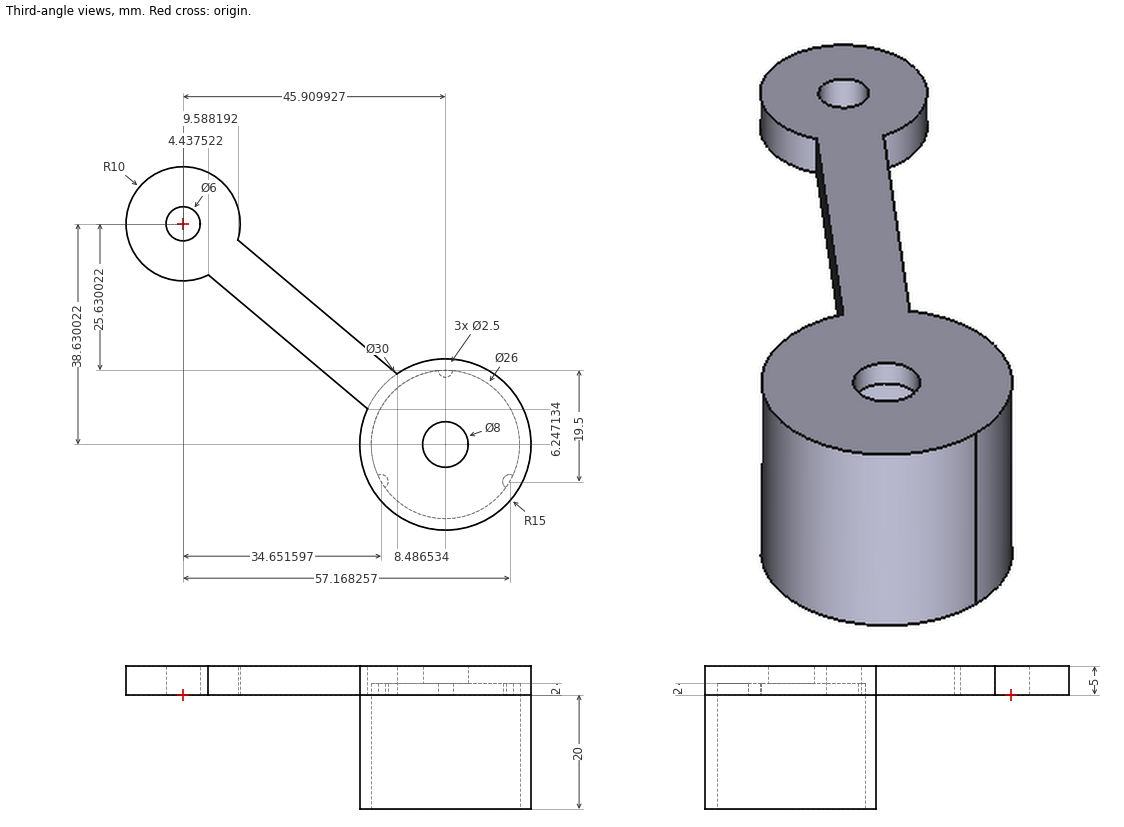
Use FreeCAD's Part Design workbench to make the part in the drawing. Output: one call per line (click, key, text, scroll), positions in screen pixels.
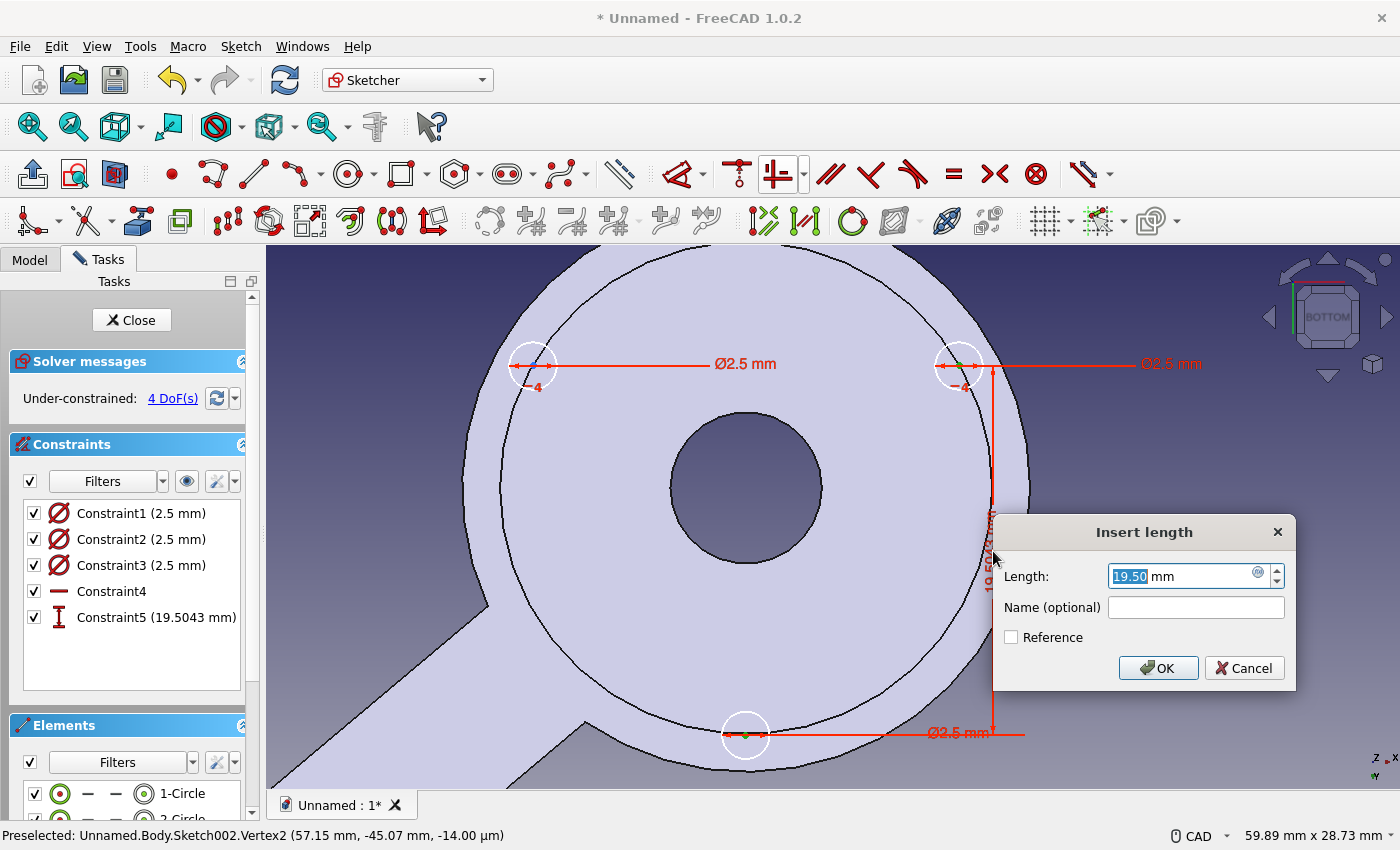
text(19.5)
key(Return)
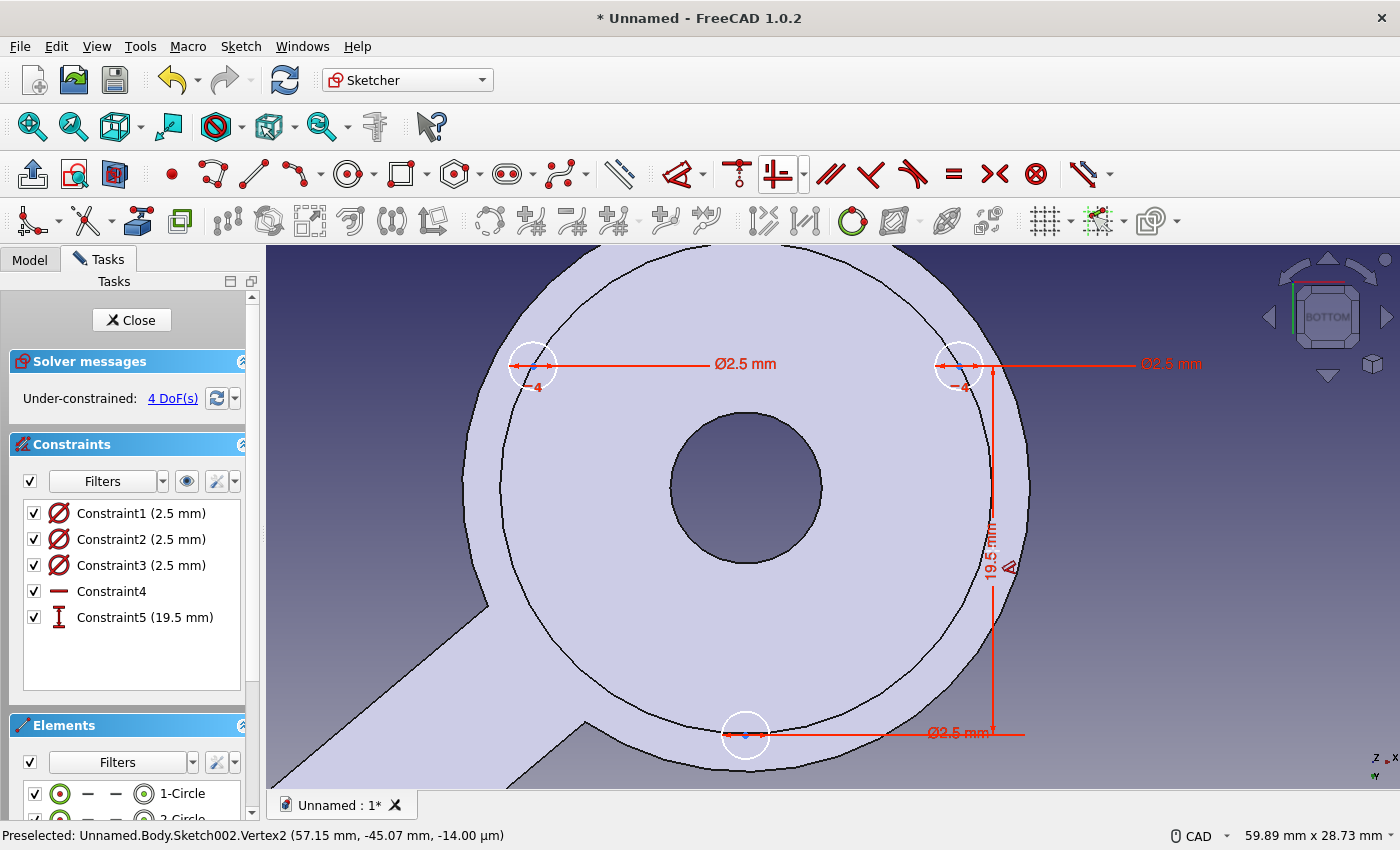
click(746, 735)
click(520, 701)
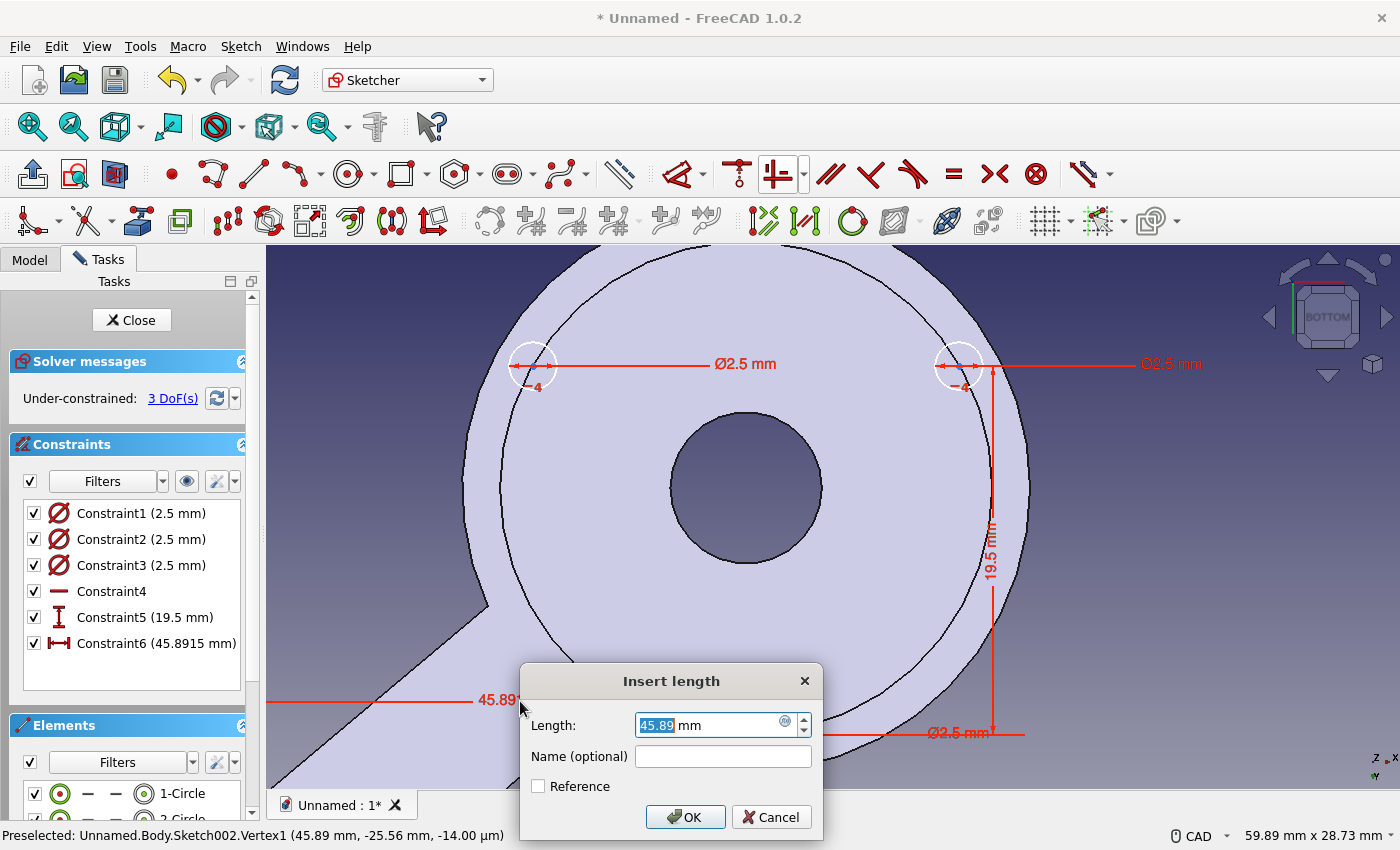
text(45.909927)
key(Return)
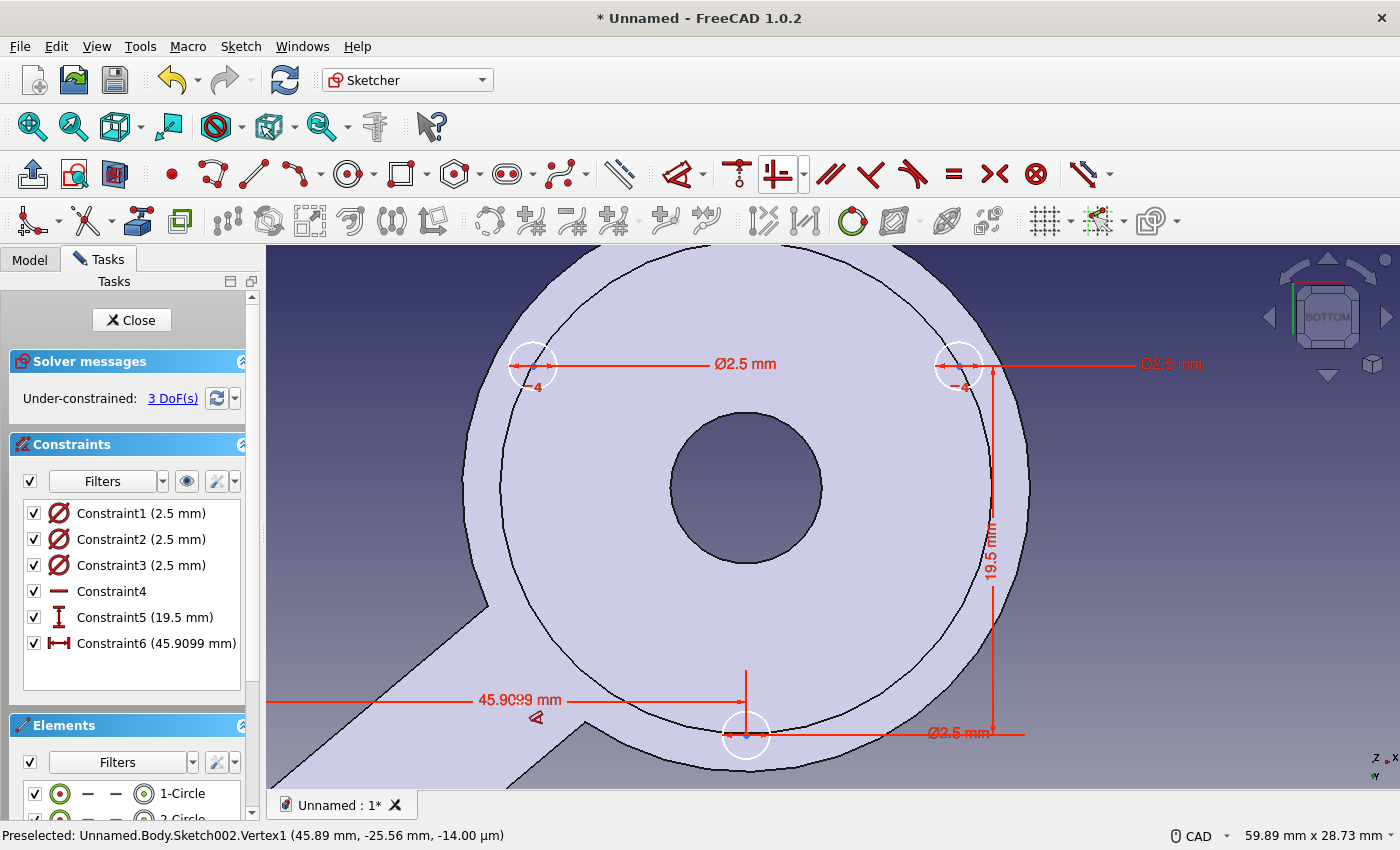
click(746, 735)
click(780, 754)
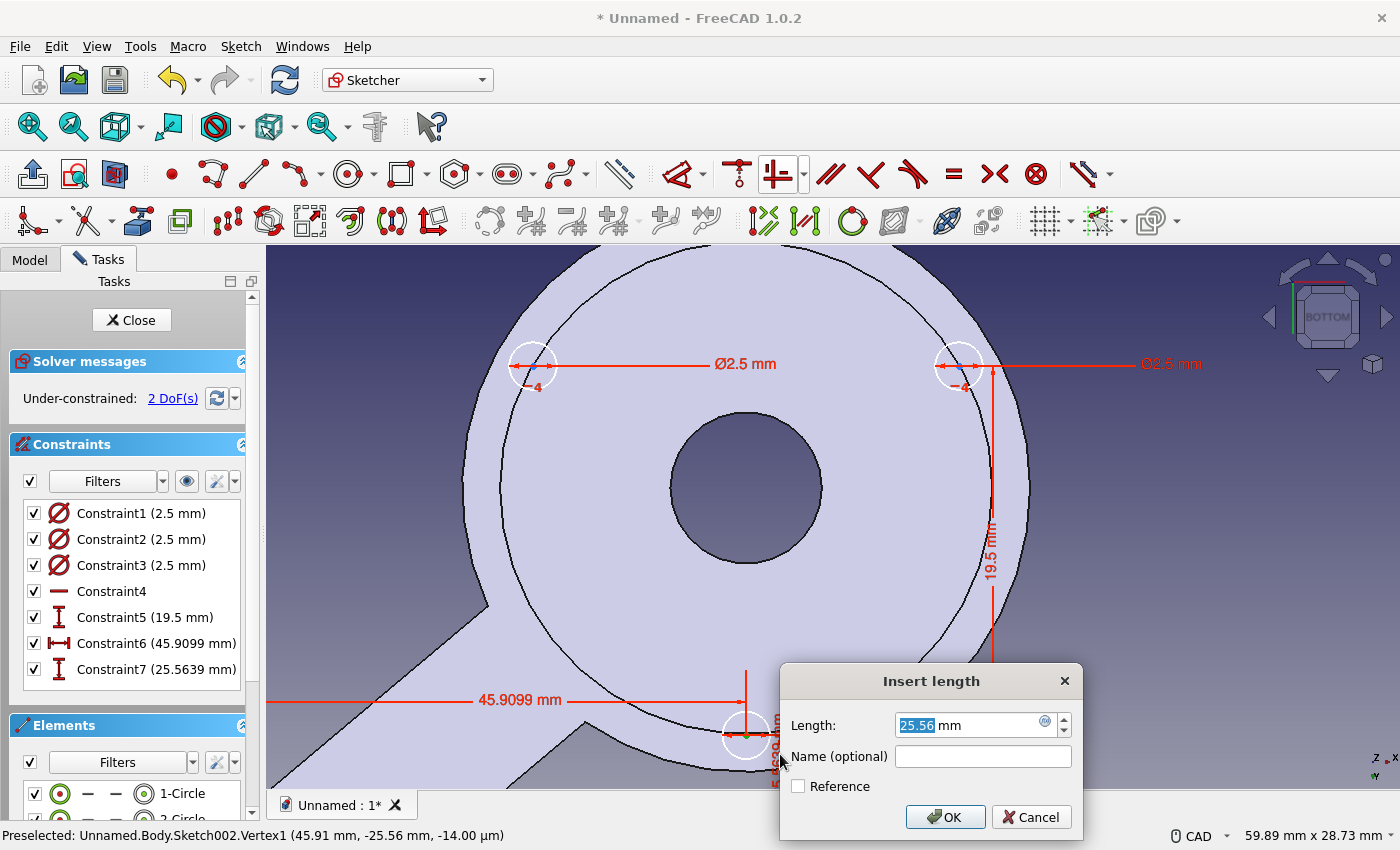
text(25.630022)
key(Return)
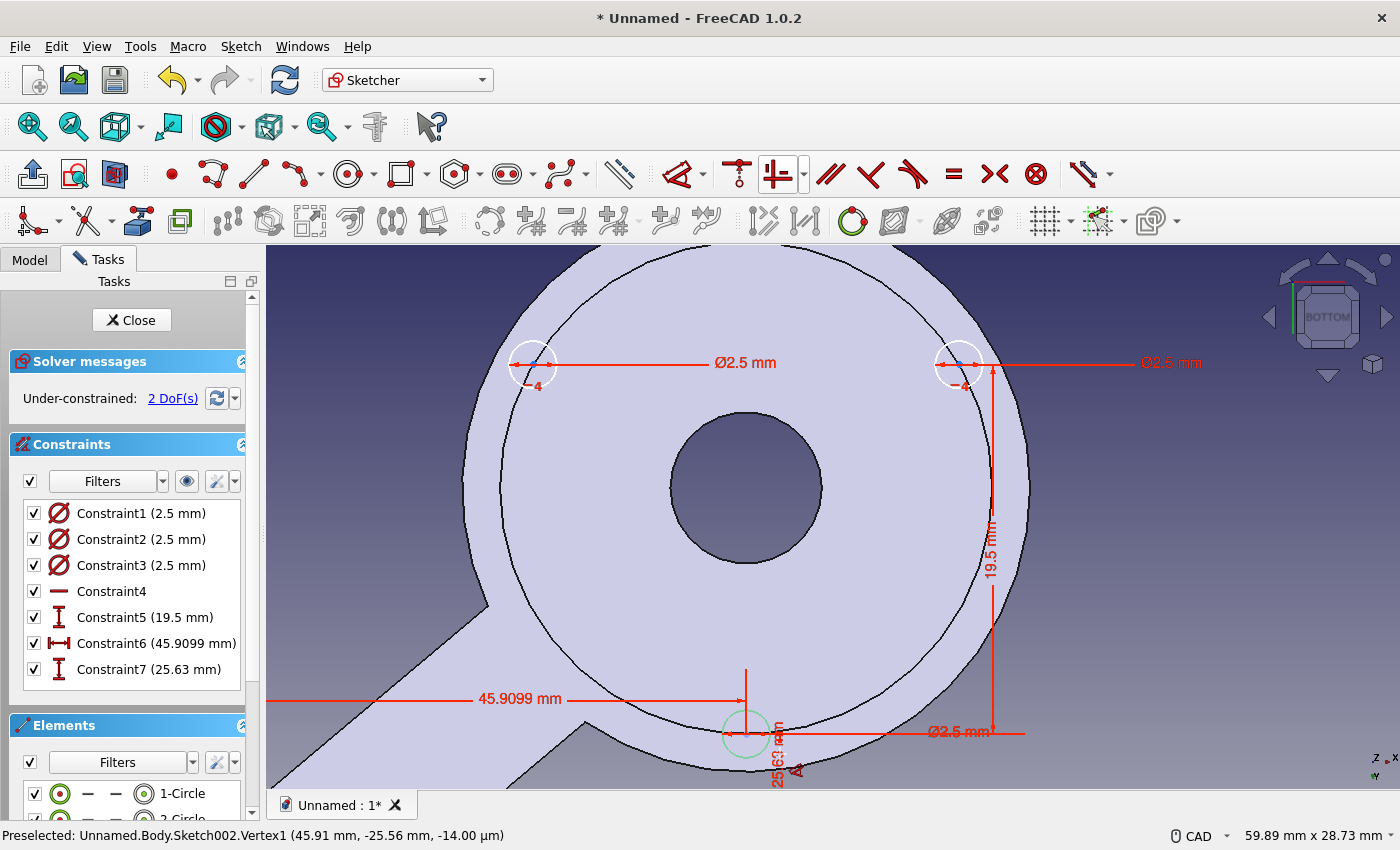
click(959, 365)
click(626, 331)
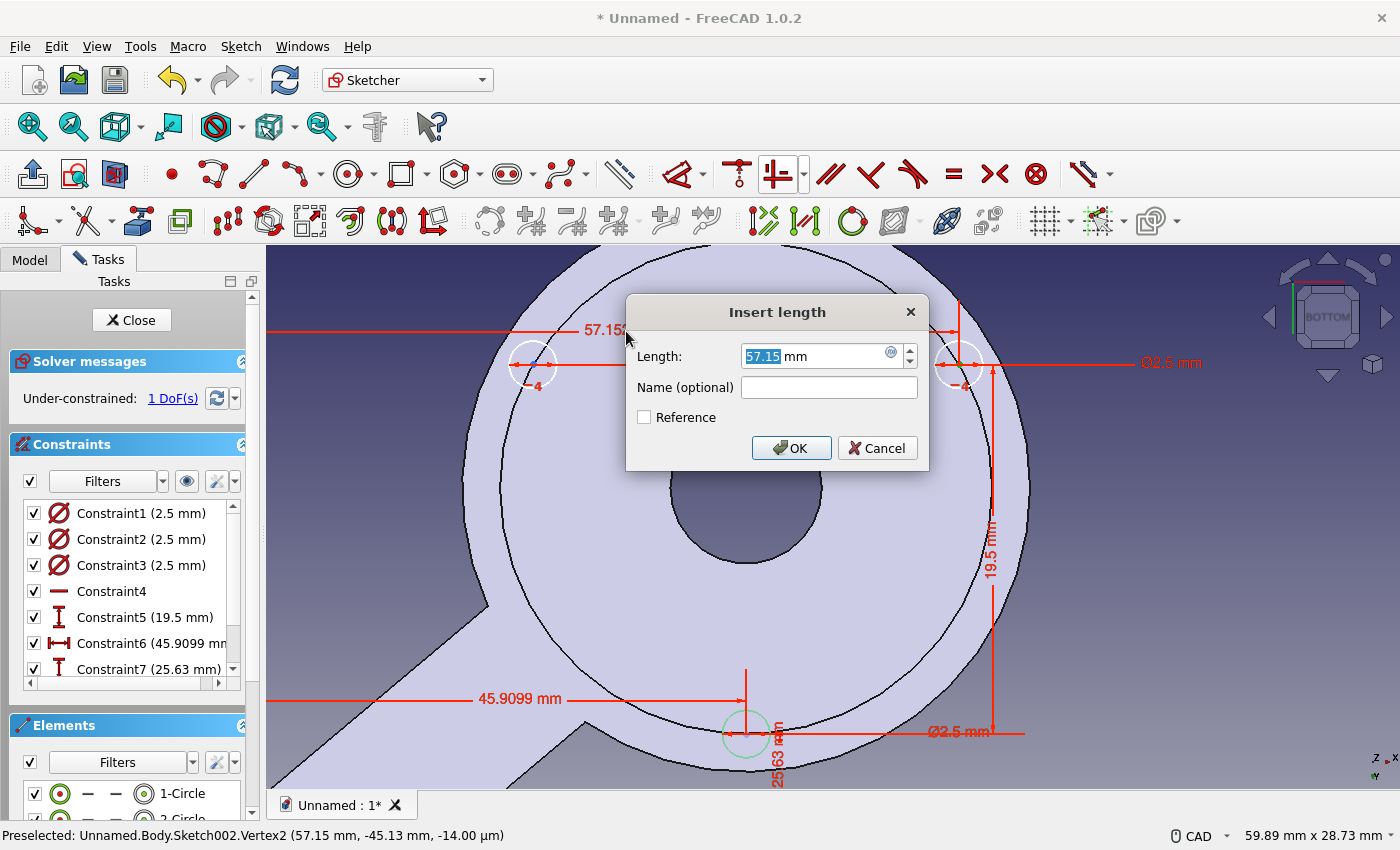
text(57.168257)
key(Return)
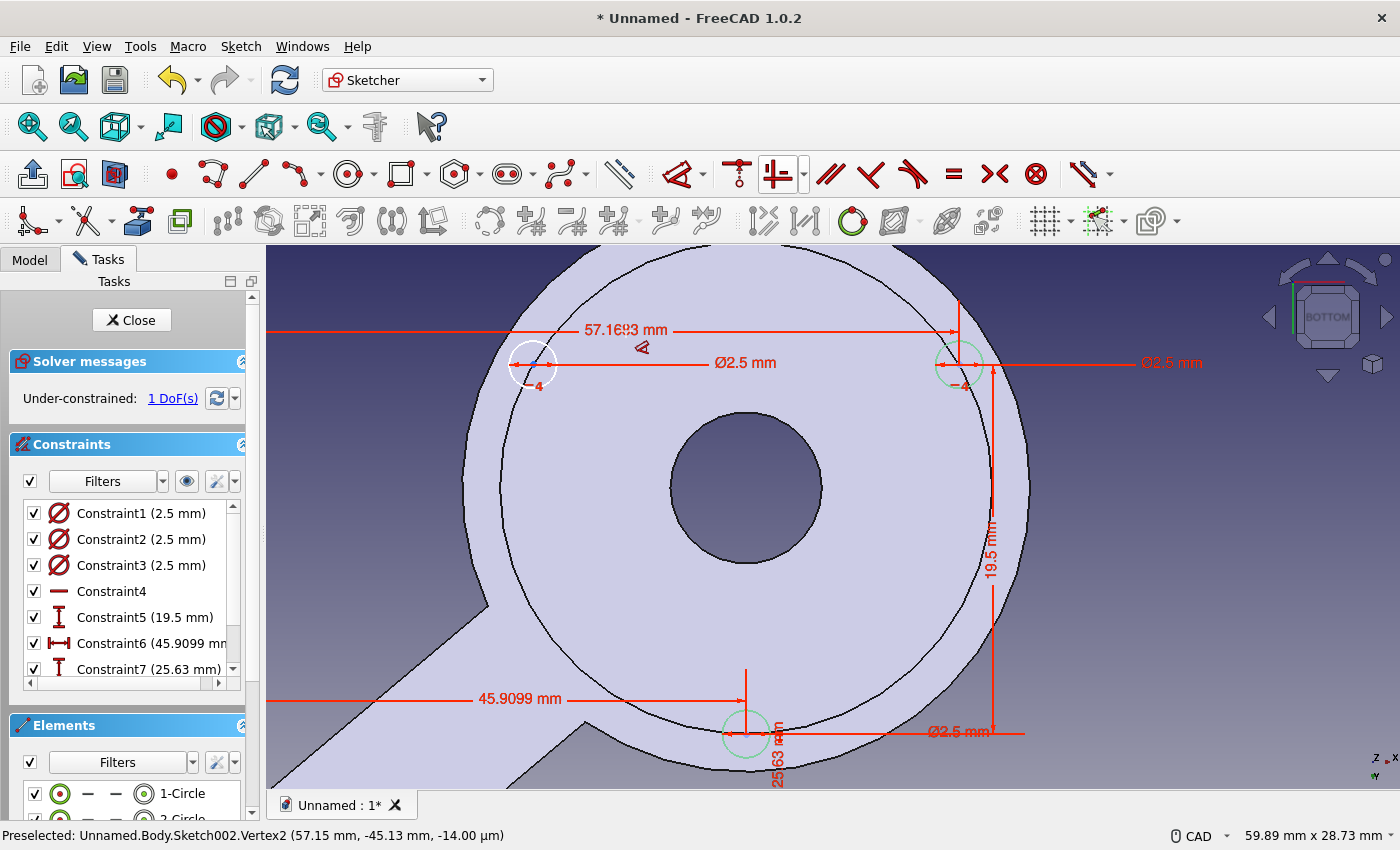
click(533, 365)
click(413, 331)